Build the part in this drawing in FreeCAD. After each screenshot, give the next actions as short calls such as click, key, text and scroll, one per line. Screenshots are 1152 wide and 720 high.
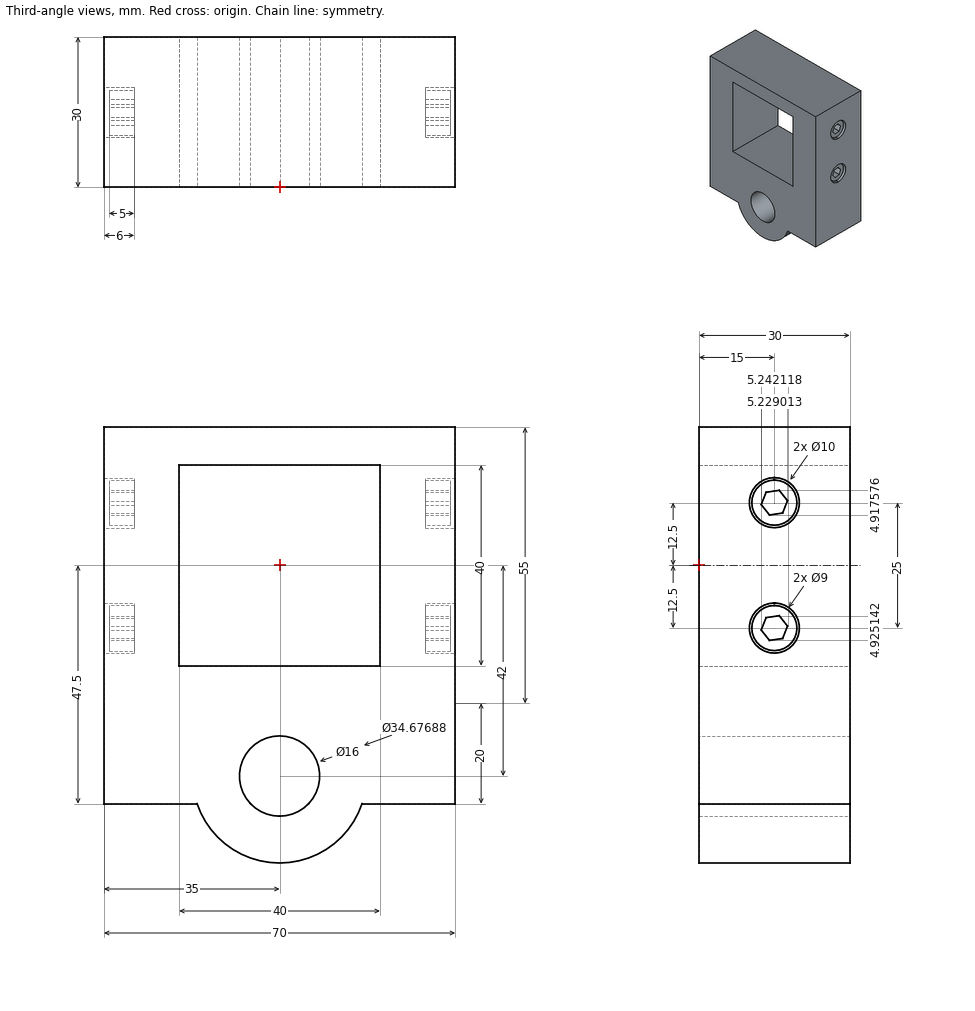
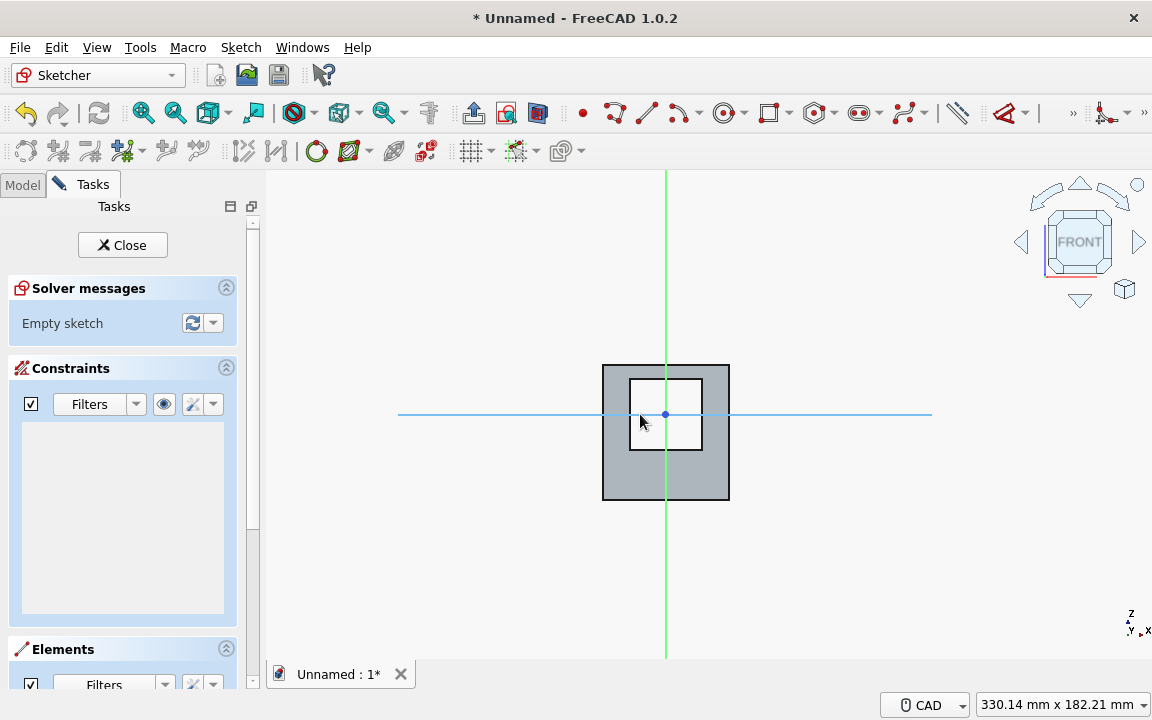
scroll(668, 498, up, 12)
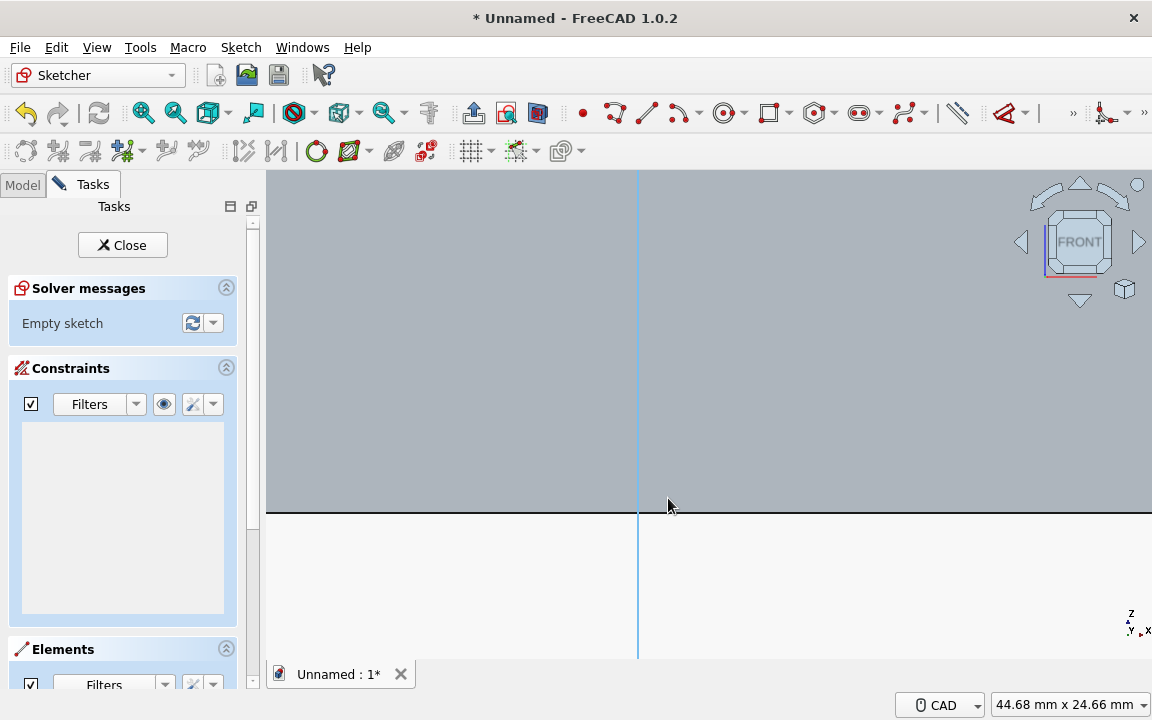
click(724, 114)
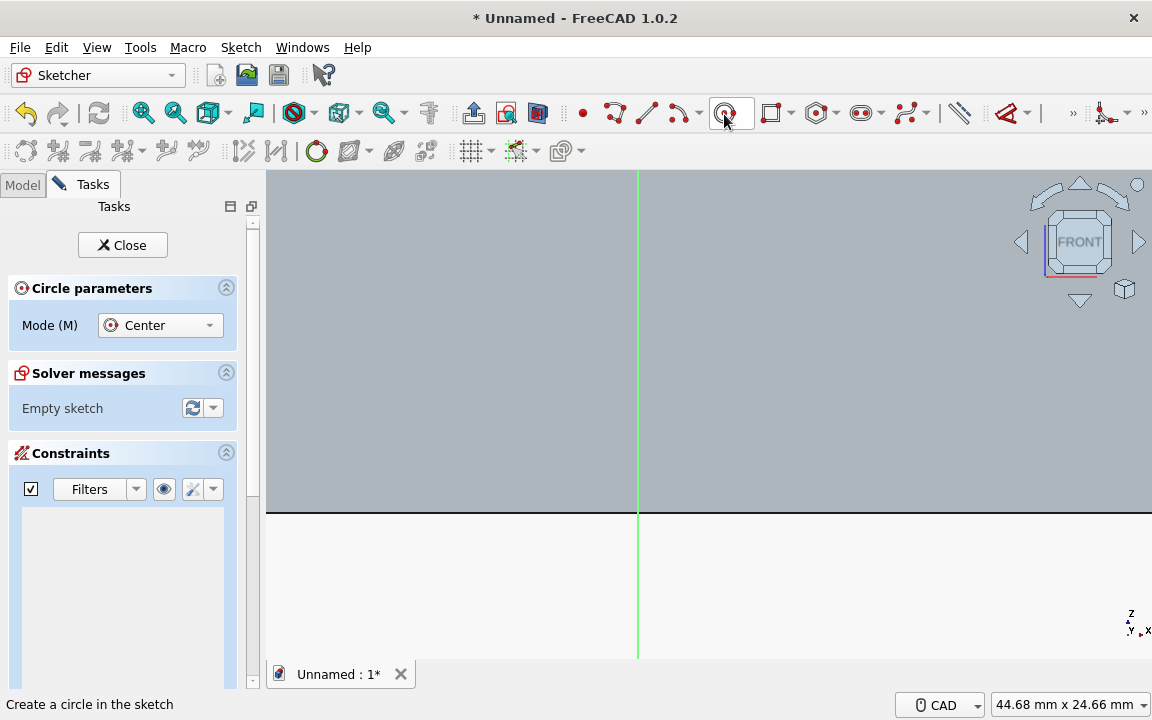
click(638, 404)
move(750, 292)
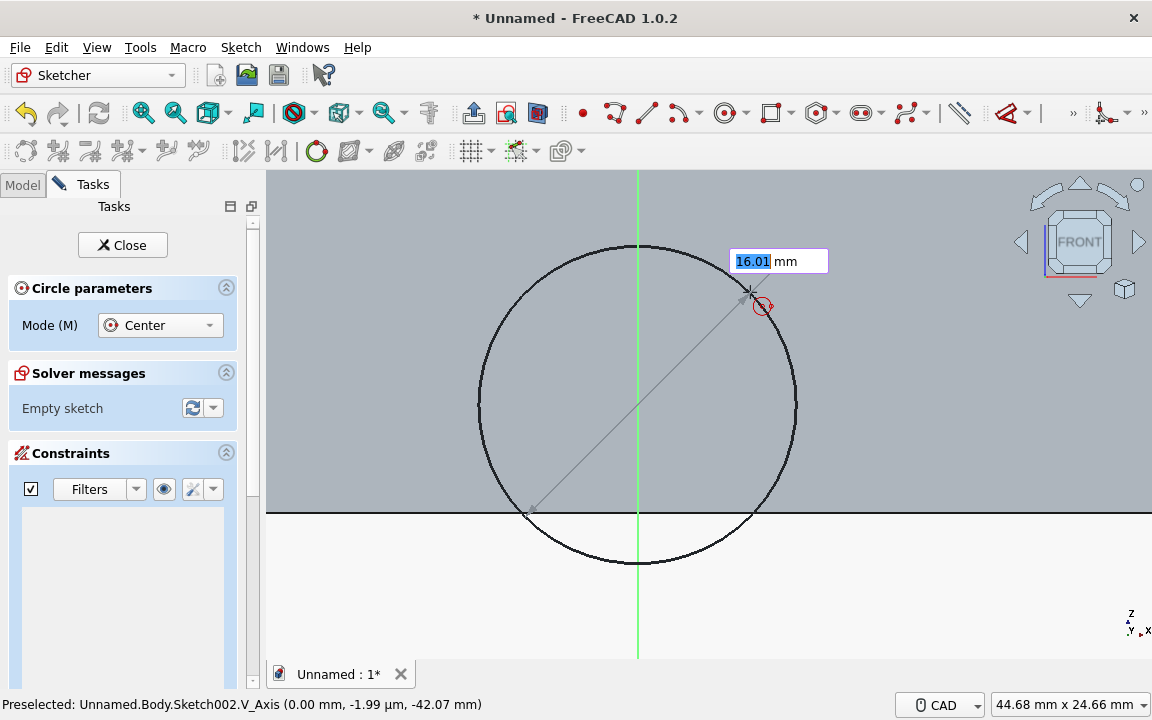
text(16)
key(Return)
key(Escape)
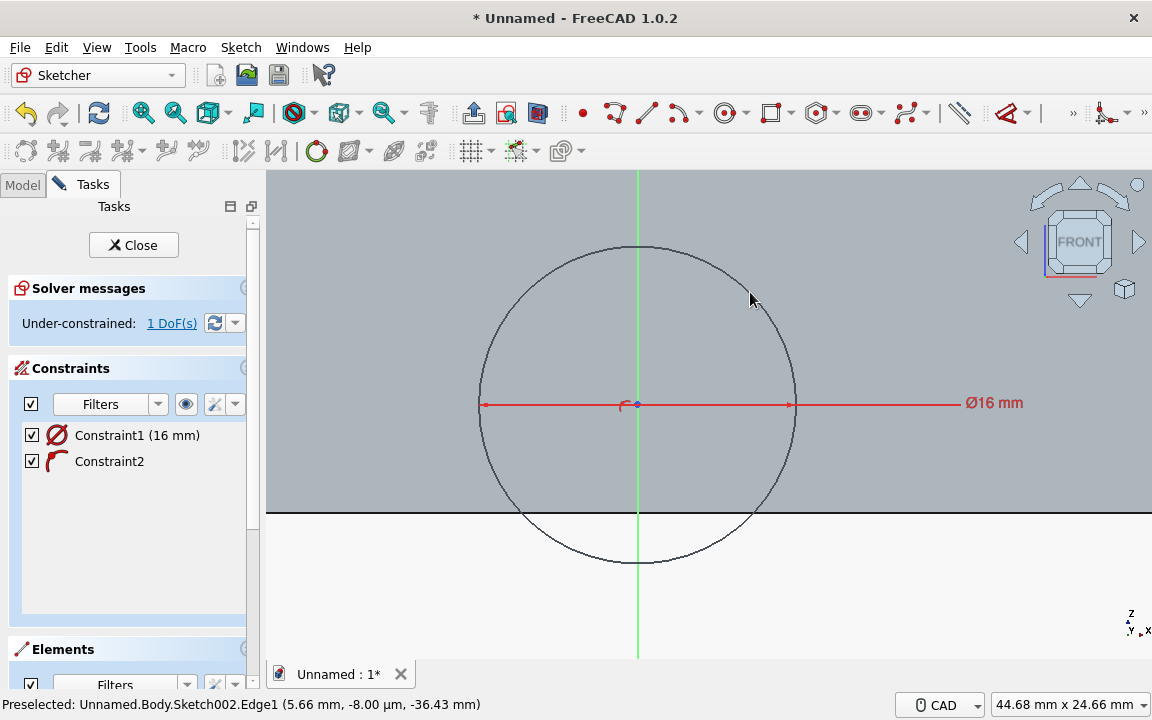
click(1006, 114)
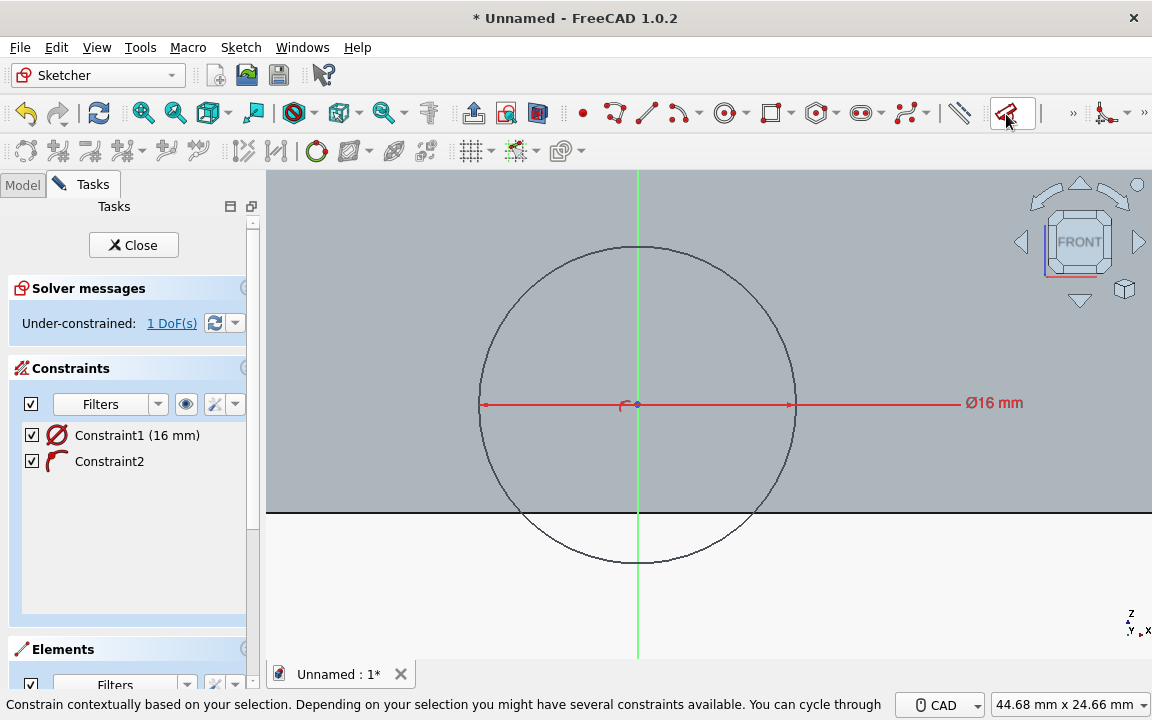
click(638, 405)
click(672, 302)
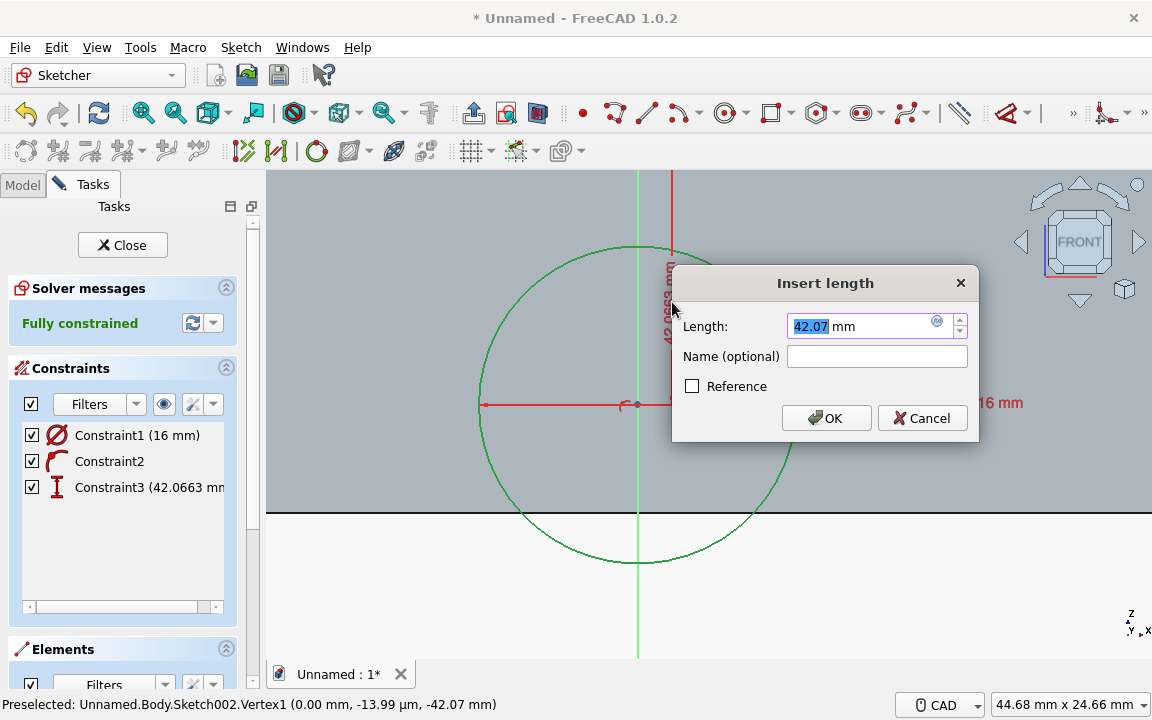
text(42)
key(Return)
key(Escape)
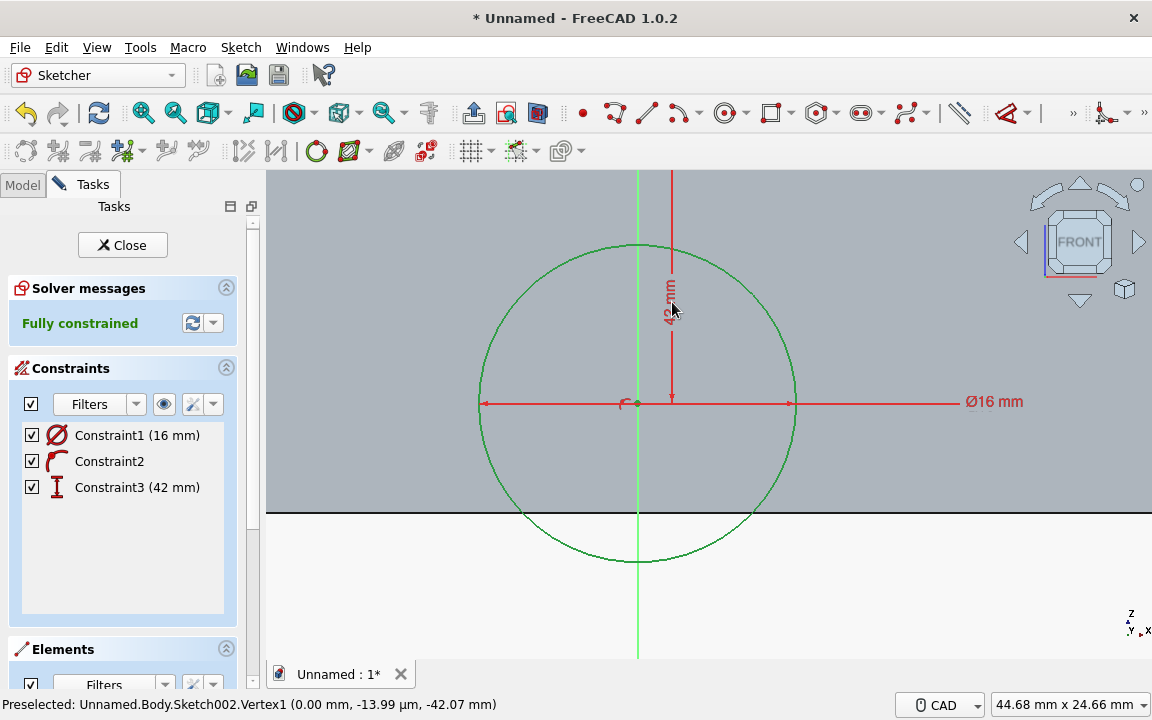
click(123, 245)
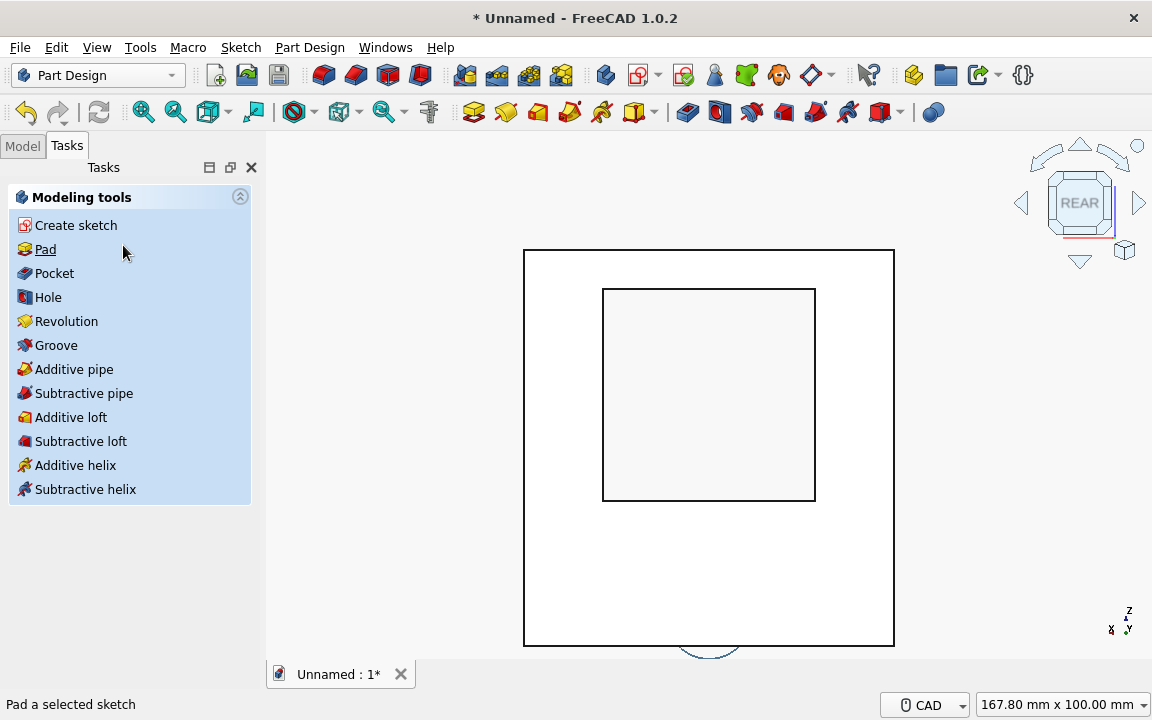
click(688, 112)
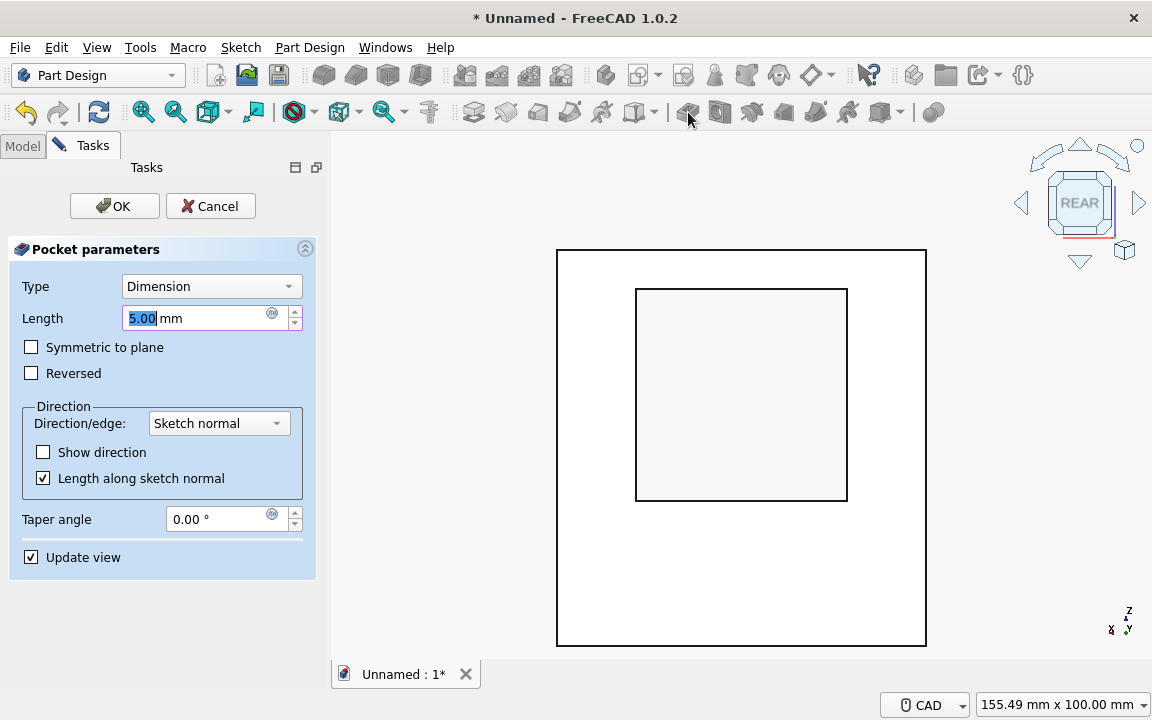
text(30)
key(Tab)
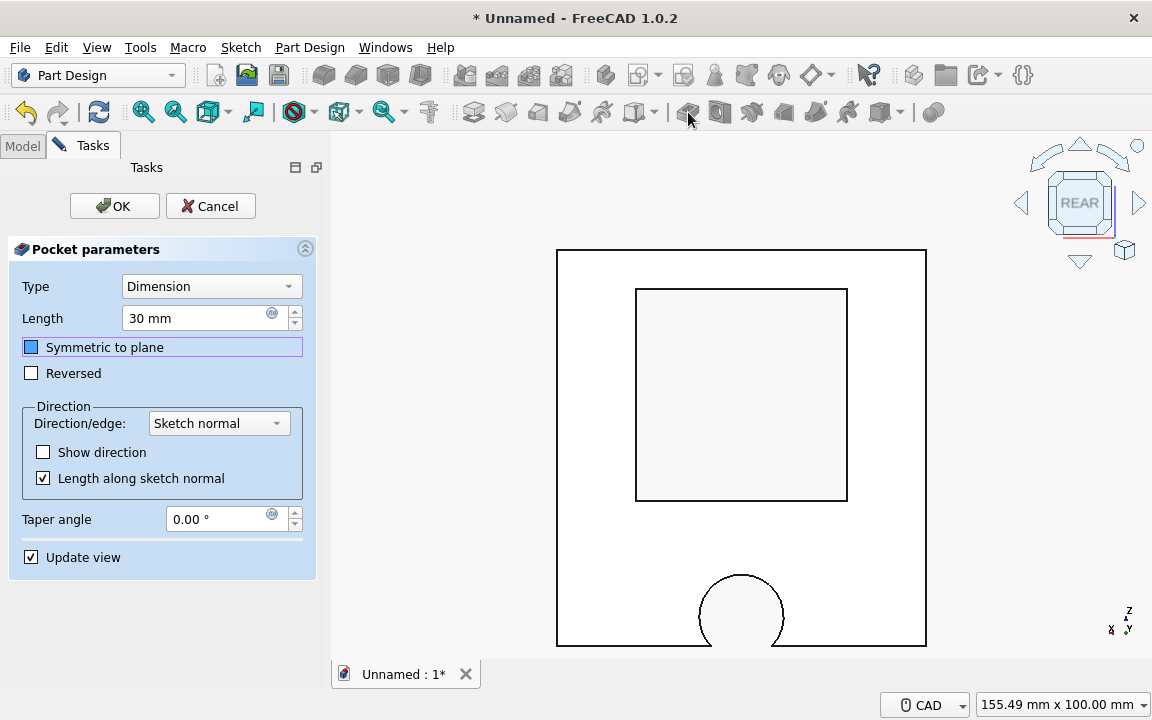
click(115, 206)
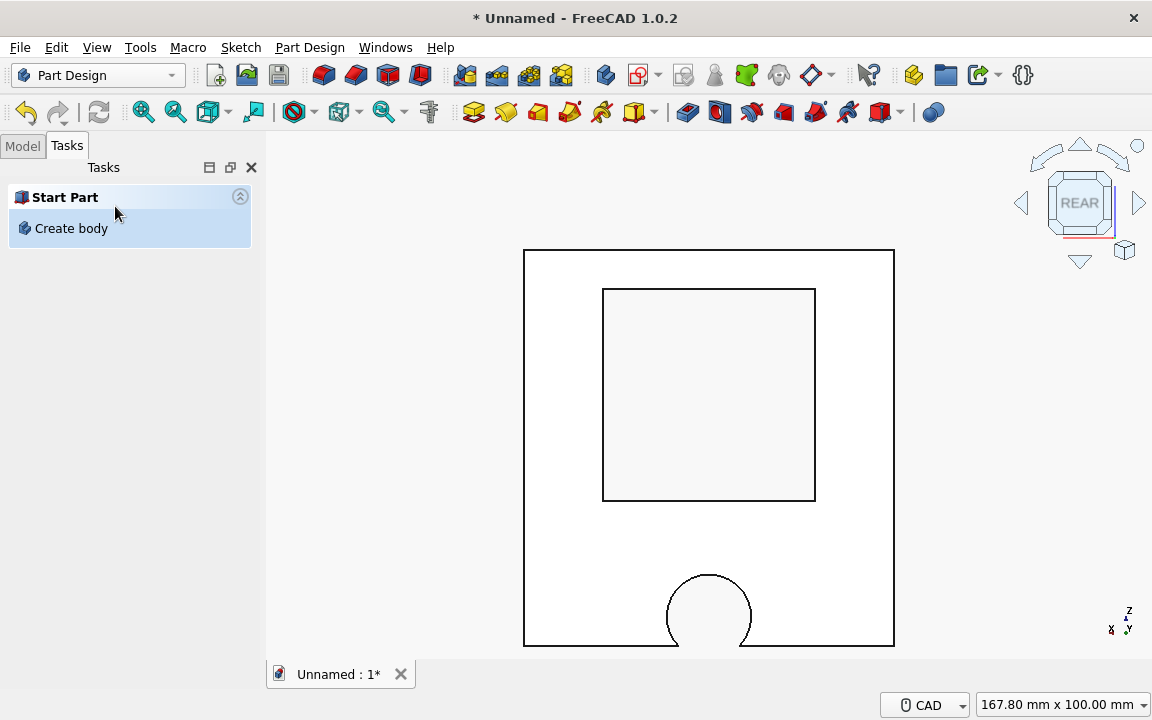
key(0)